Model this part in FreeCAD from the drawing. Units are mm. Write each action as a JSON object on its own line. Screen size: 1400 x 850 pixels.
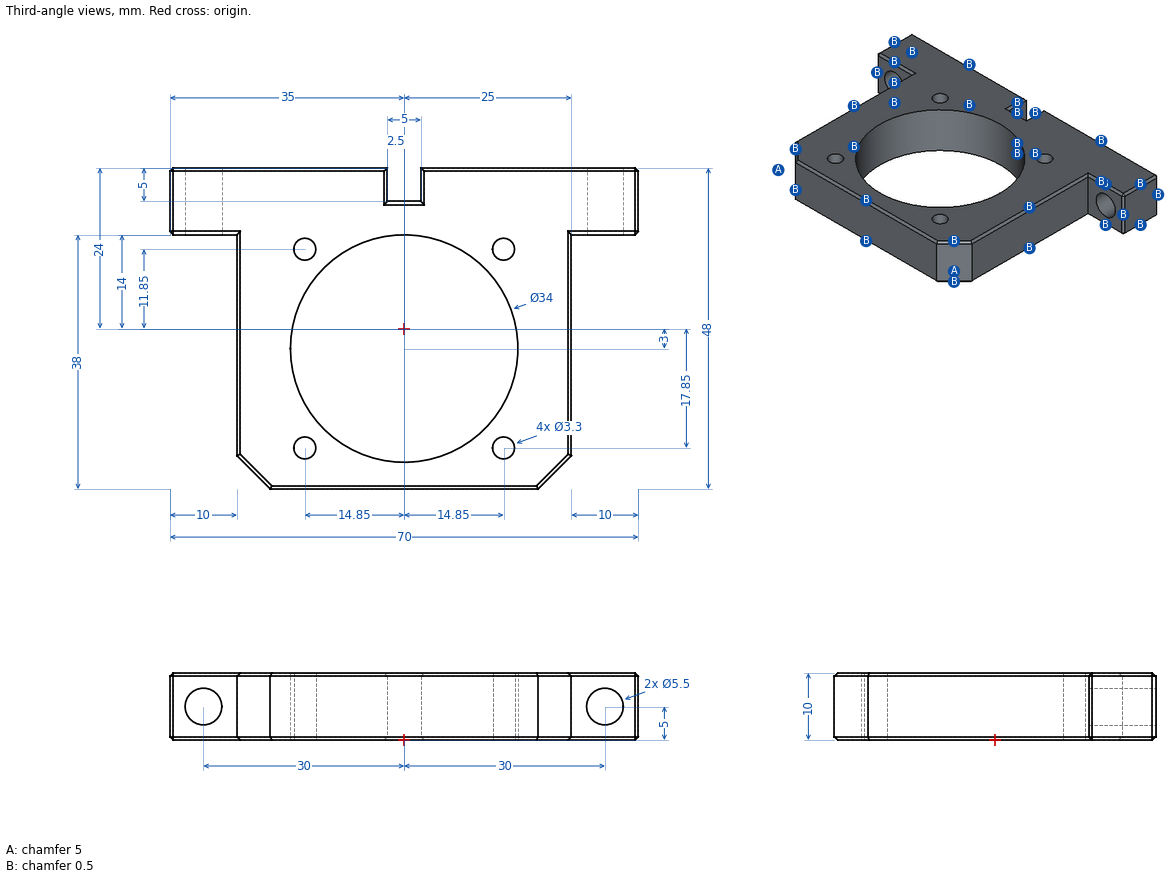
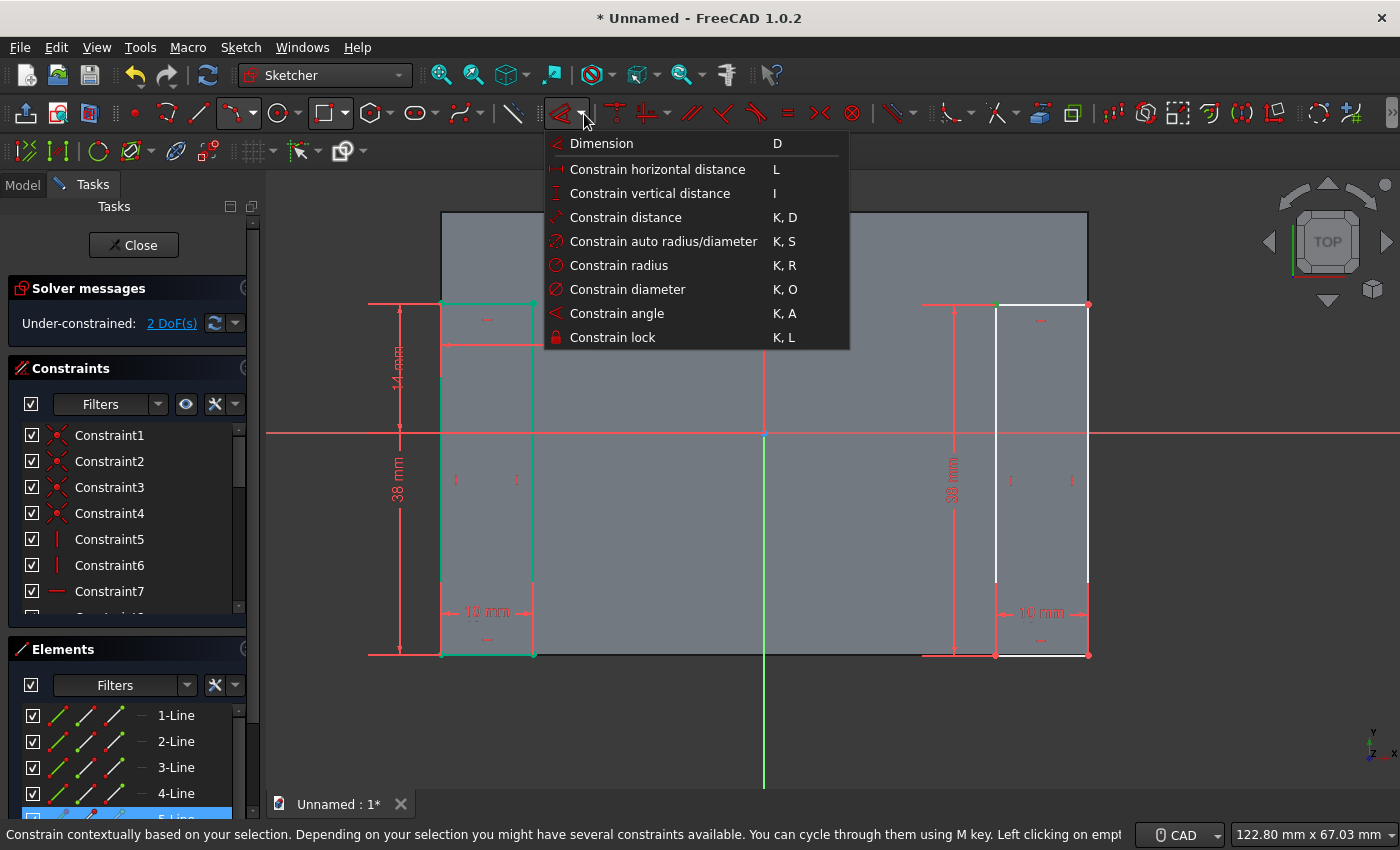
{"action": "left_click", "coordinate": [697, 169]}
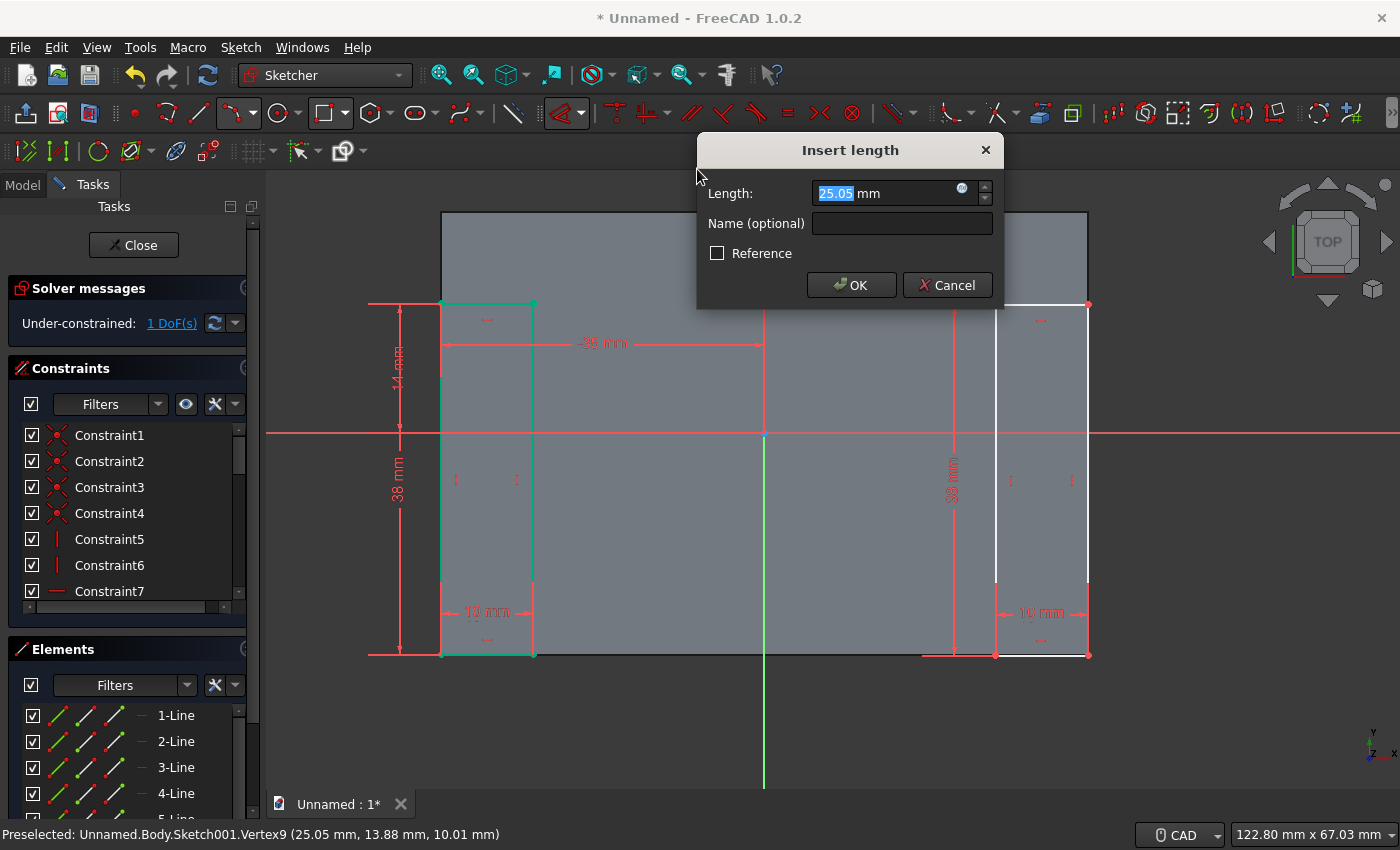
{"action": "type", "text": "25"}
{"action": "key", "text": "Return"}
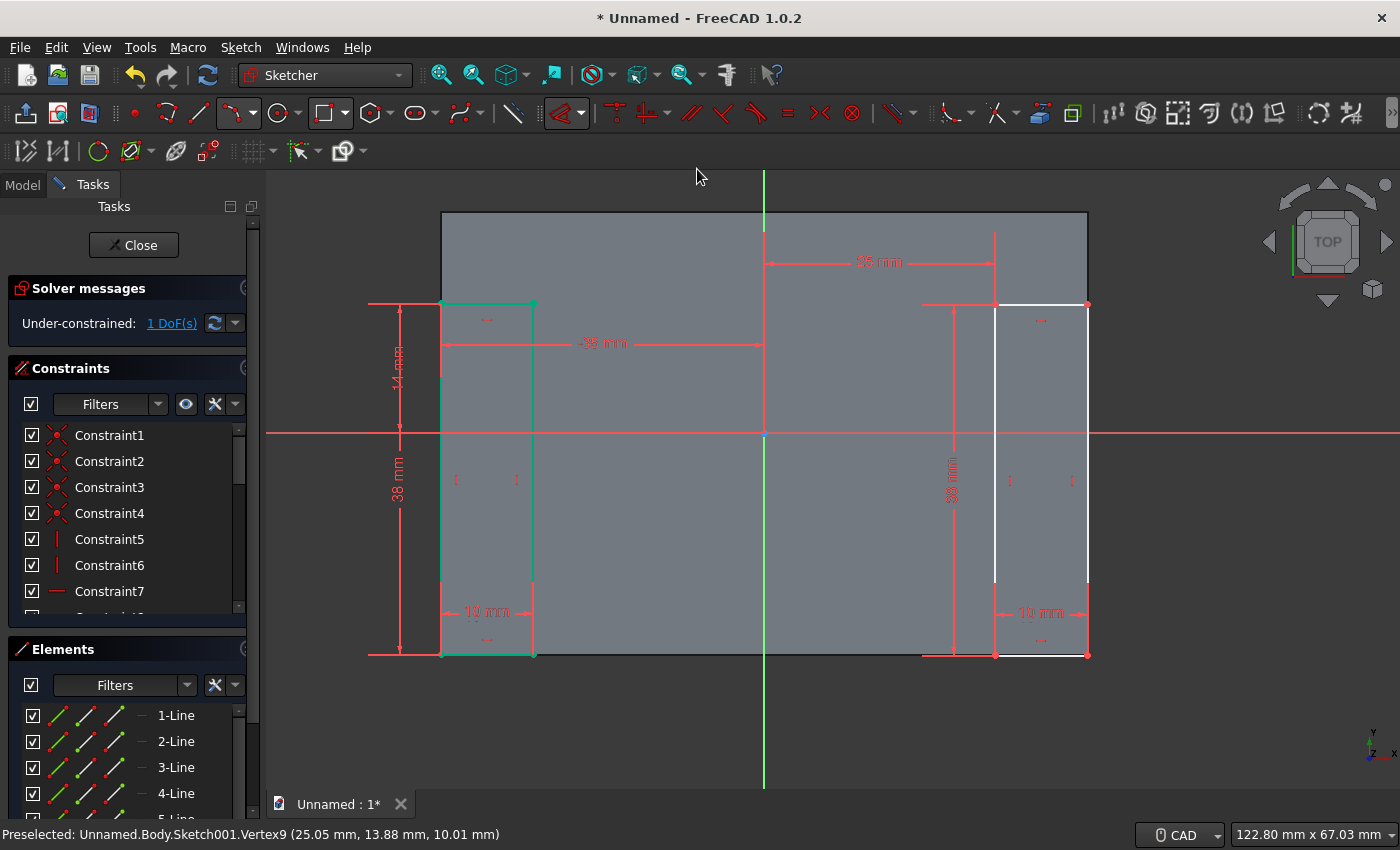
{"action": "left_click", "coordinate": [995, 305]}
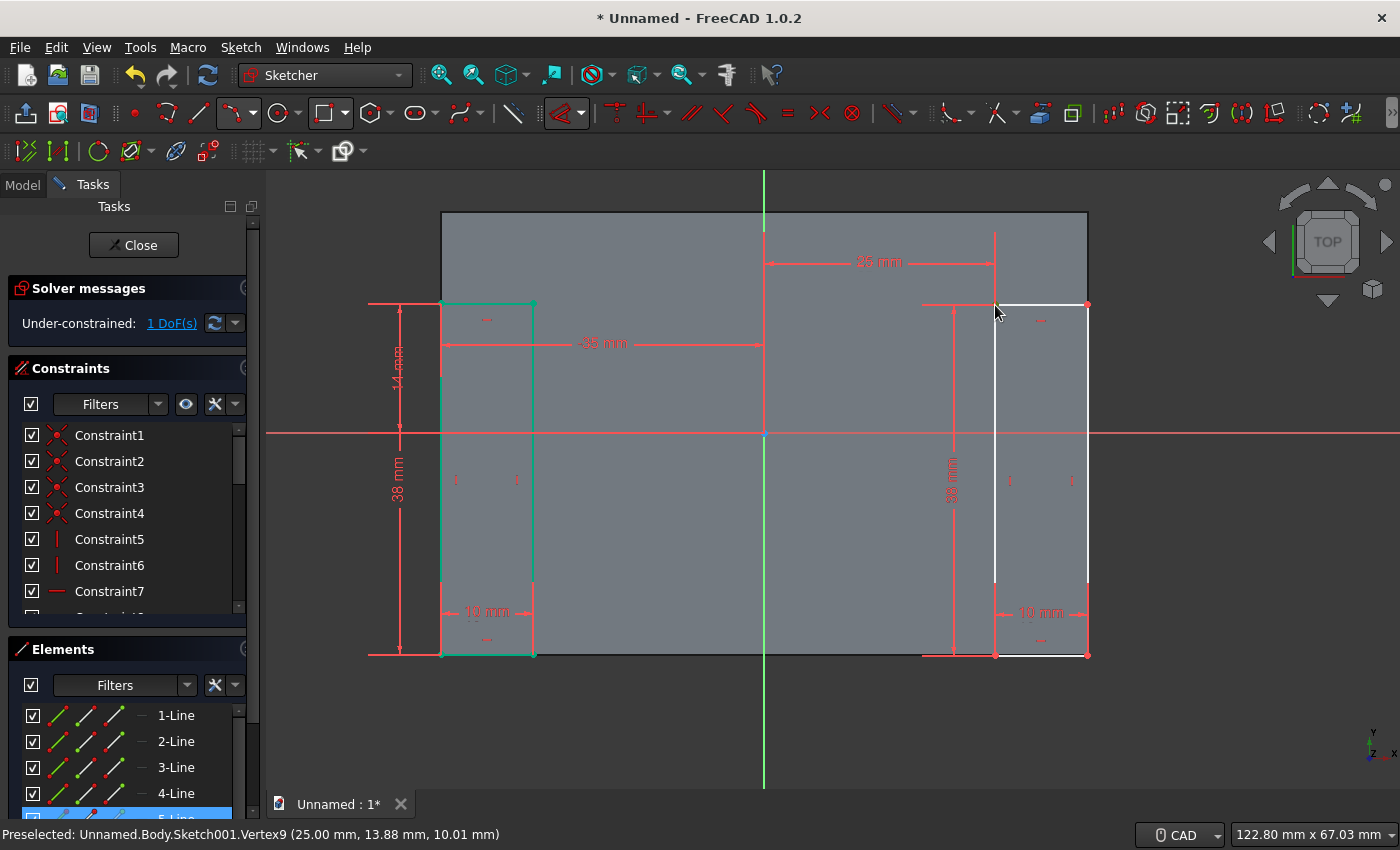
{"action": "left_click", "coordinate": [584, 114]}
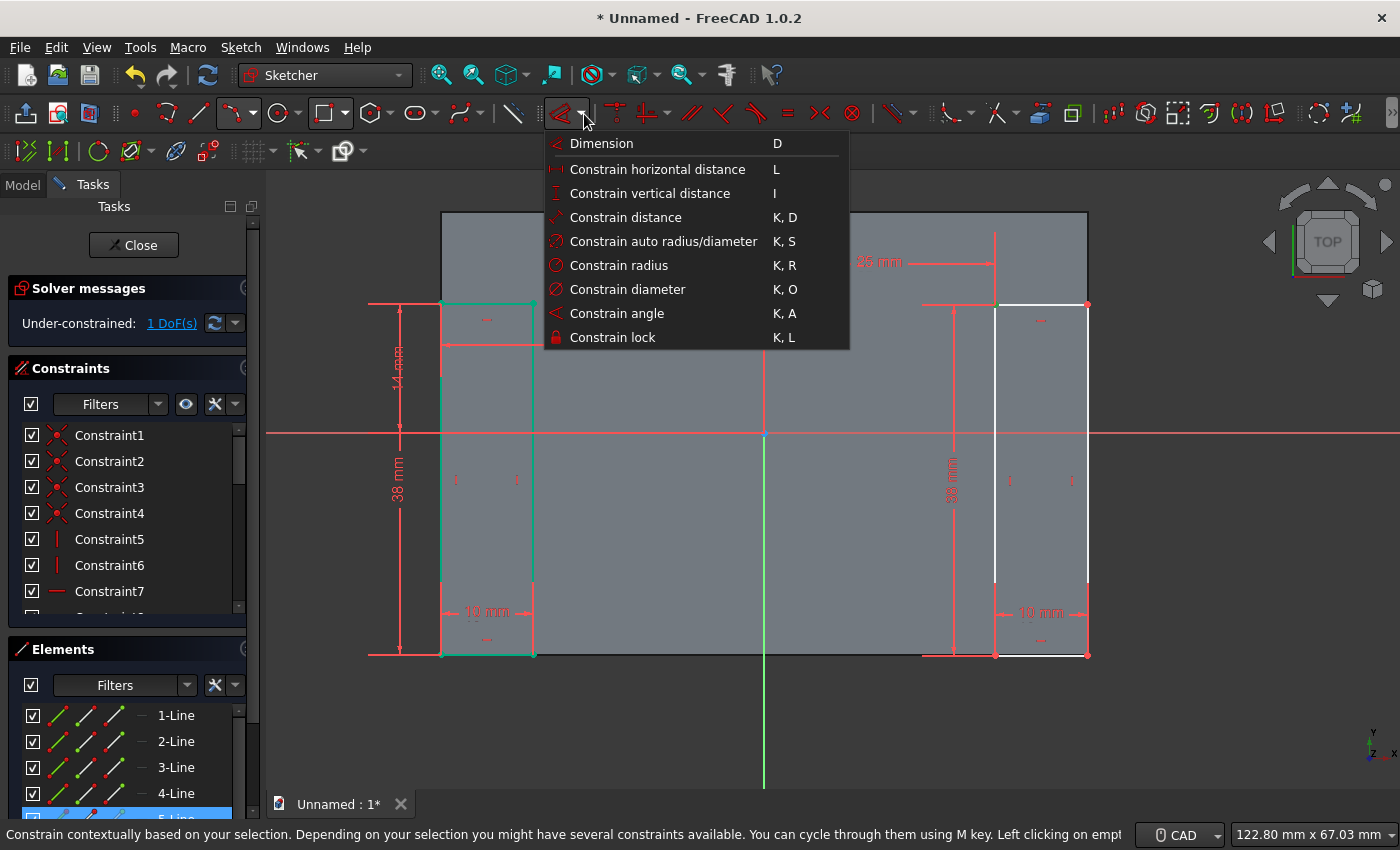
{"action": "left_click", "coordinate": [697, 193]}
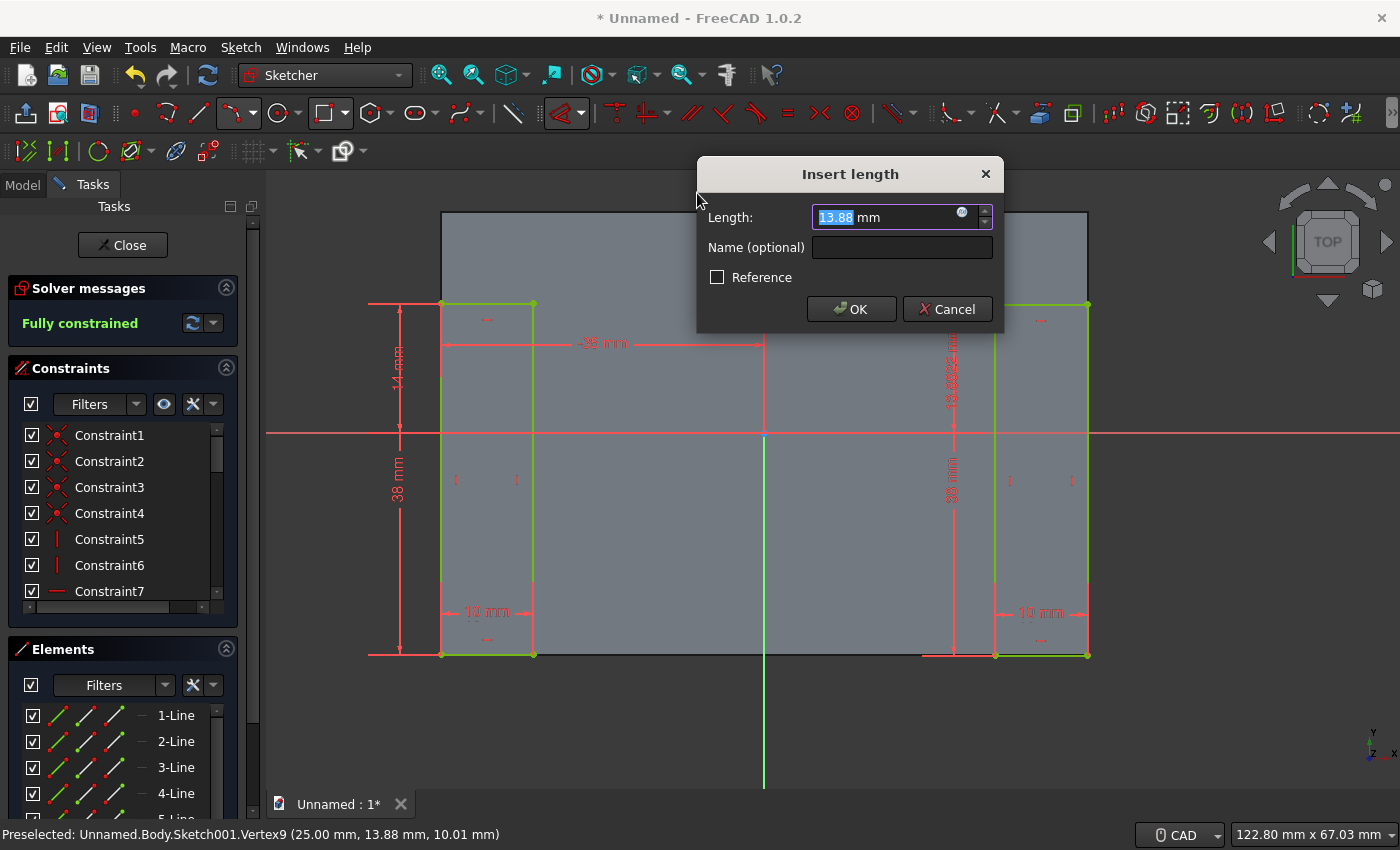
{"action": "type", "text": "14"}
{"action": "key", "text": "Return"}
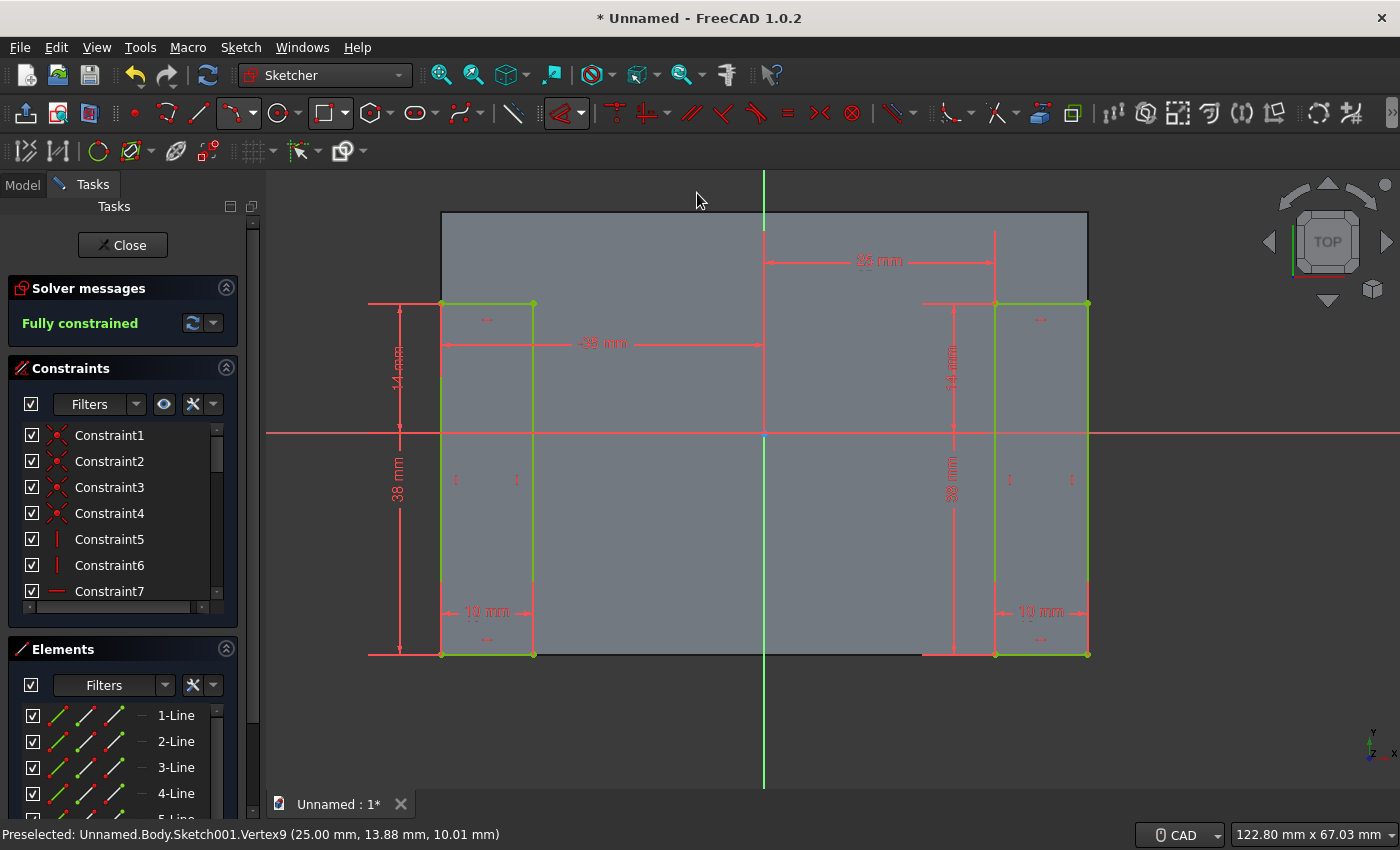
{"action": "left_click", "coordinate": [123, 245]}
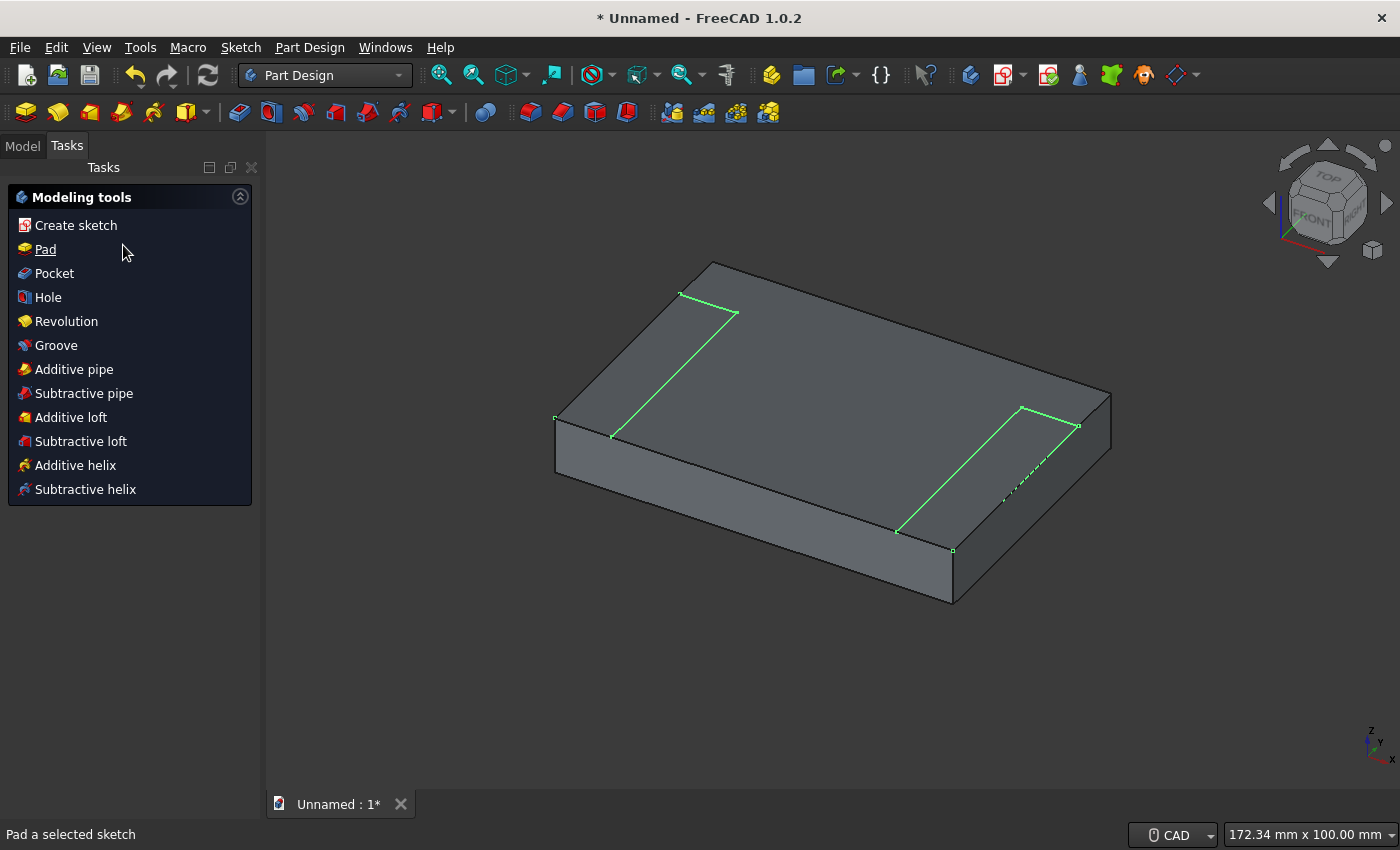
{"action": "left_click", "coordinate": [240, 112]}